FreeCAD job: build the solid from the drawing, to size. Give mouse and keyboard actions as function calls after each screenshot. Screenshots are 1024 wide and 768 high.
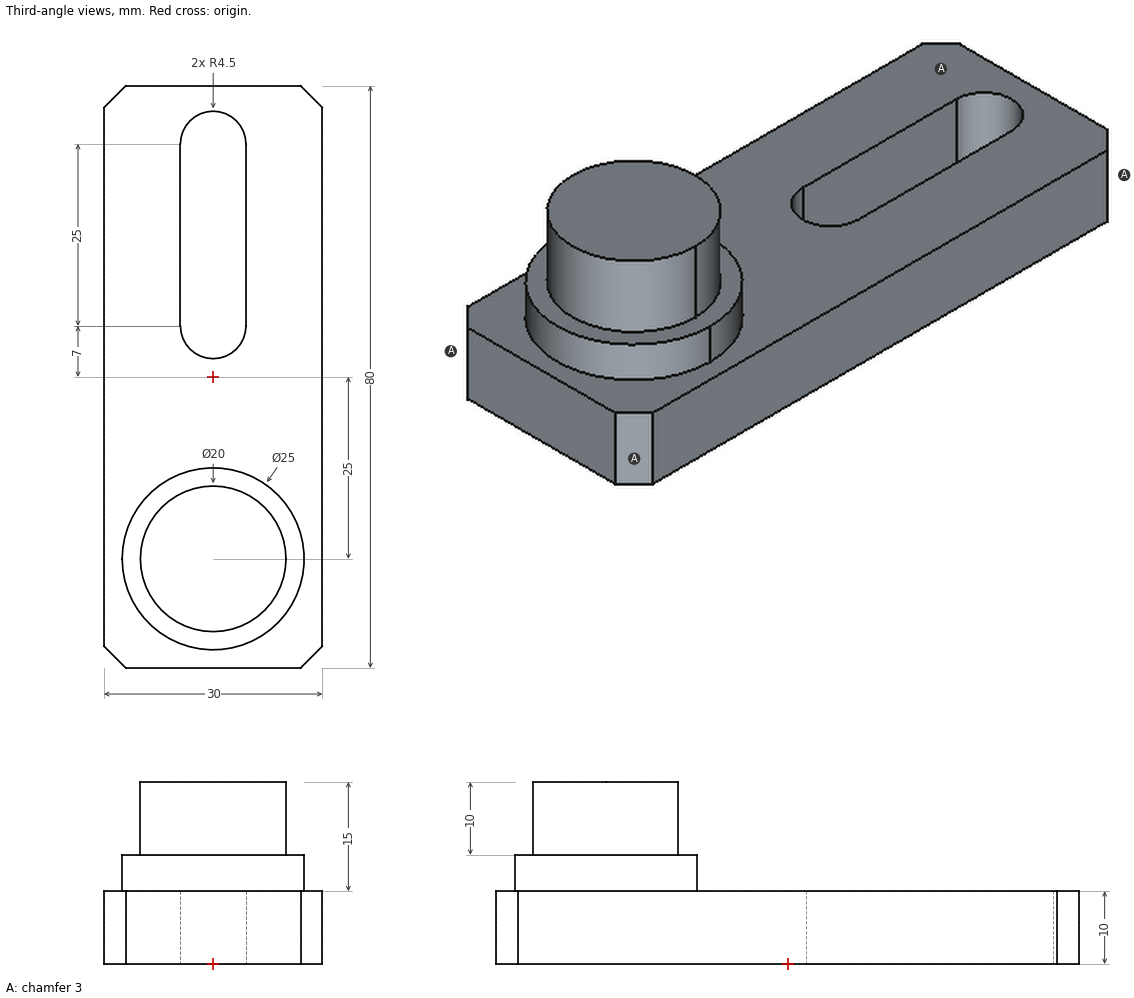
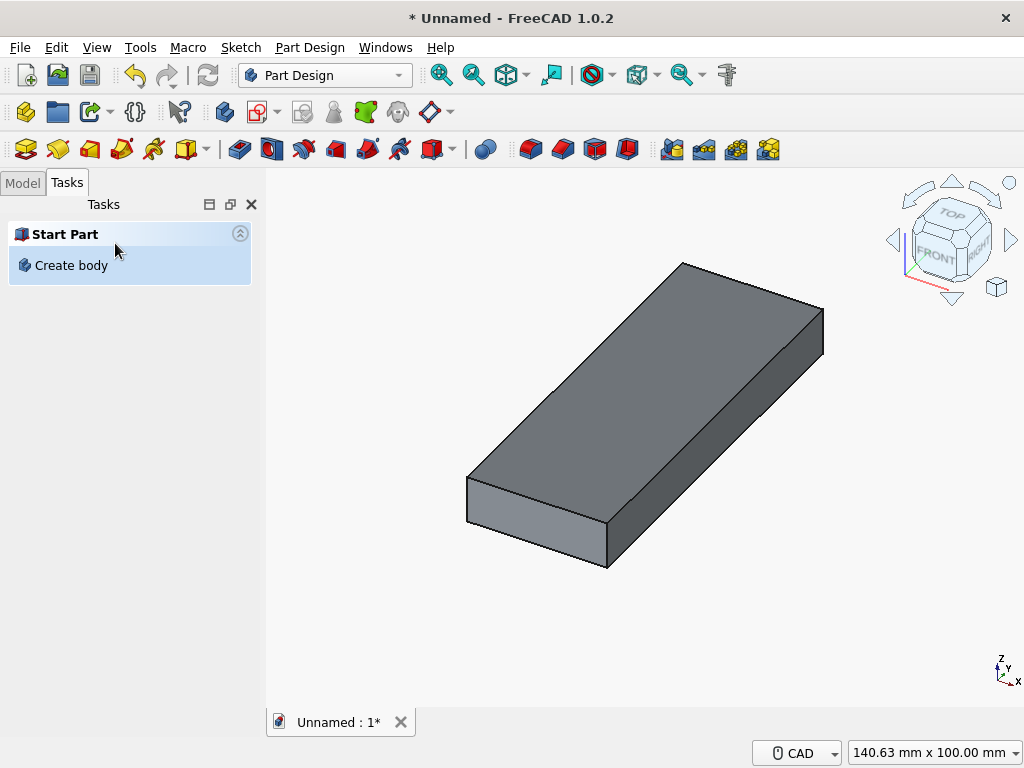
click(707, 331)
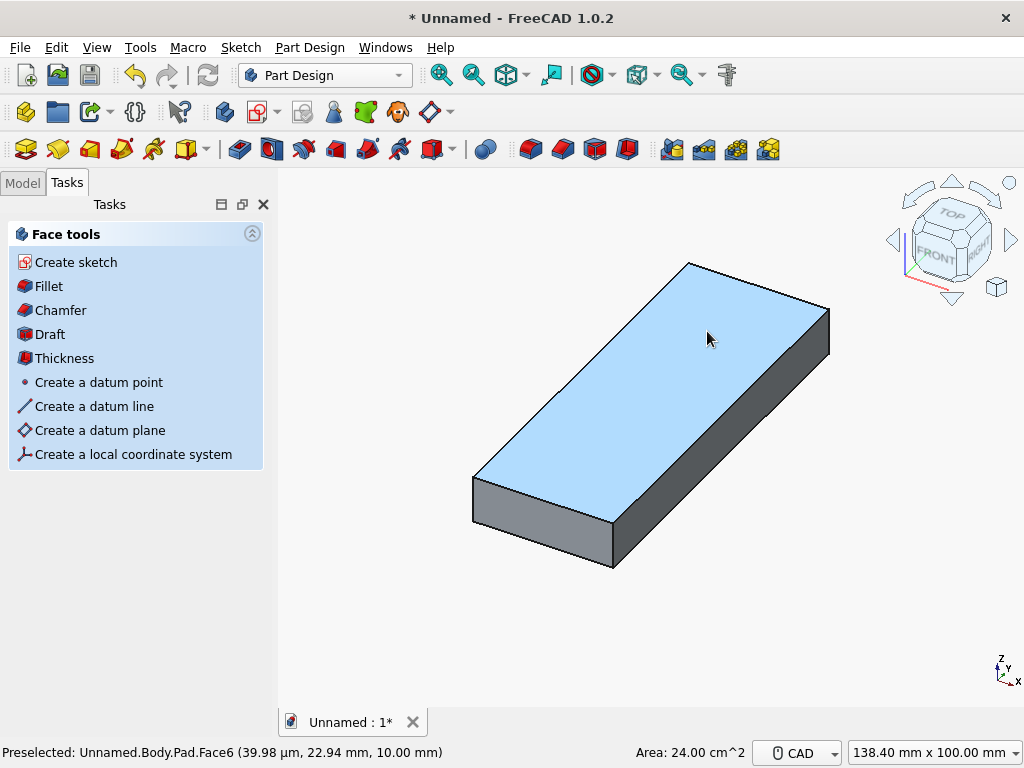
click(258, 112)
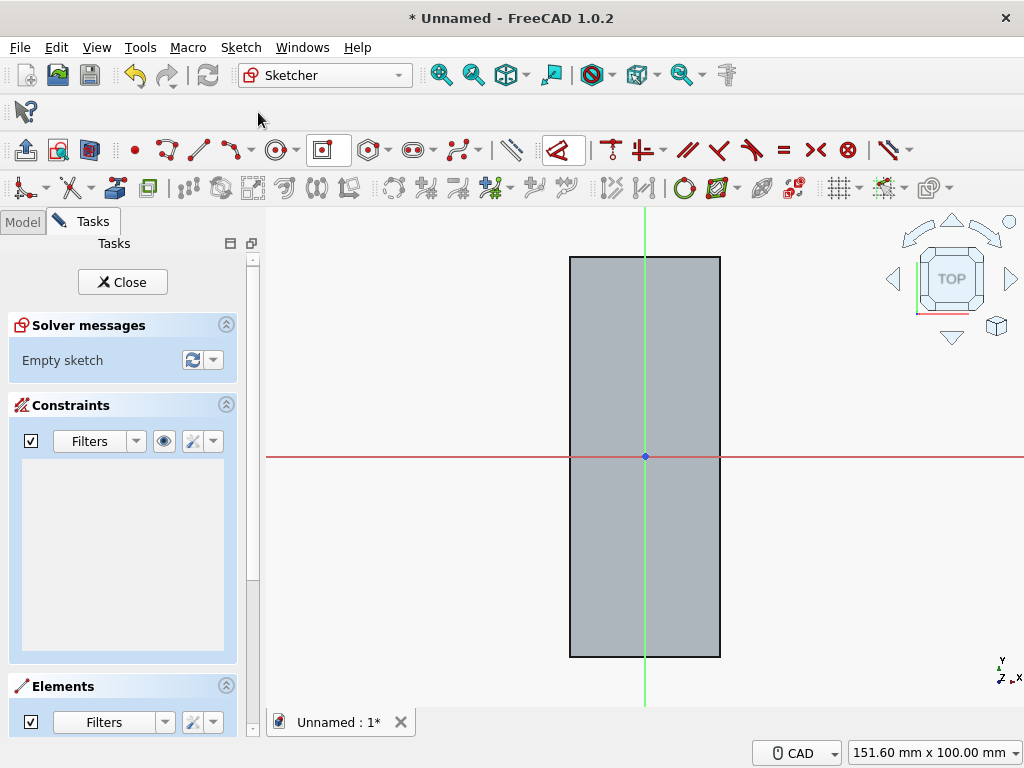
scroll(728, 665, up, 3)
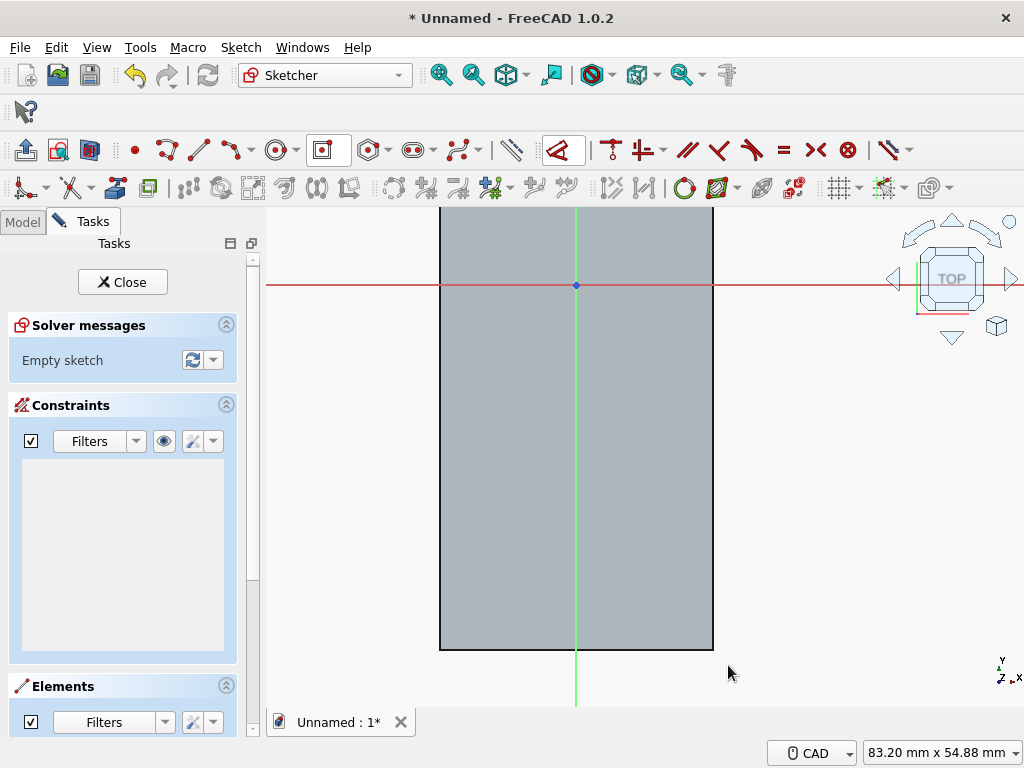
click(276, 150)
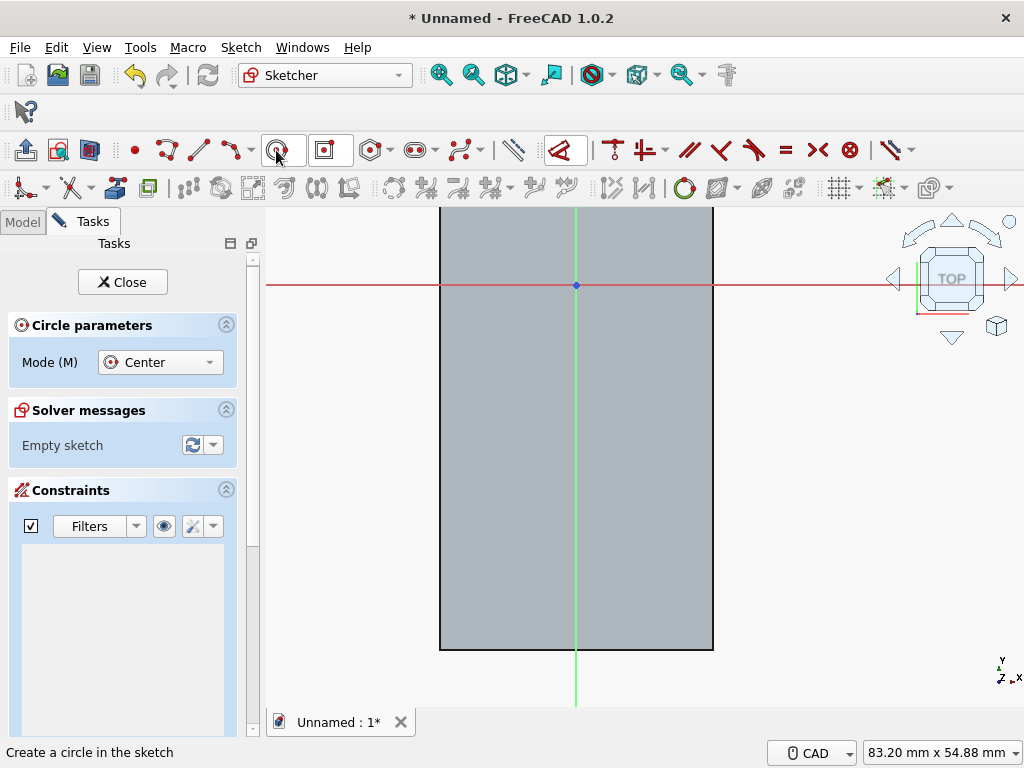
click(576, 513)
move(657, 432)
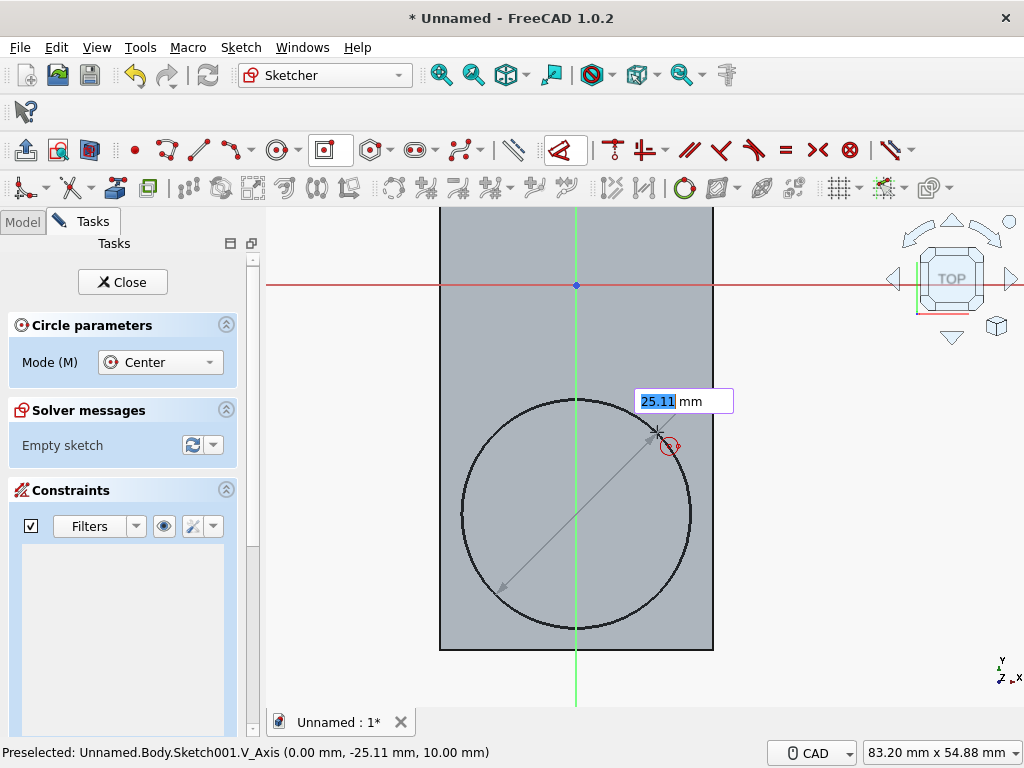
text(25)
key(Return)
key(Escape)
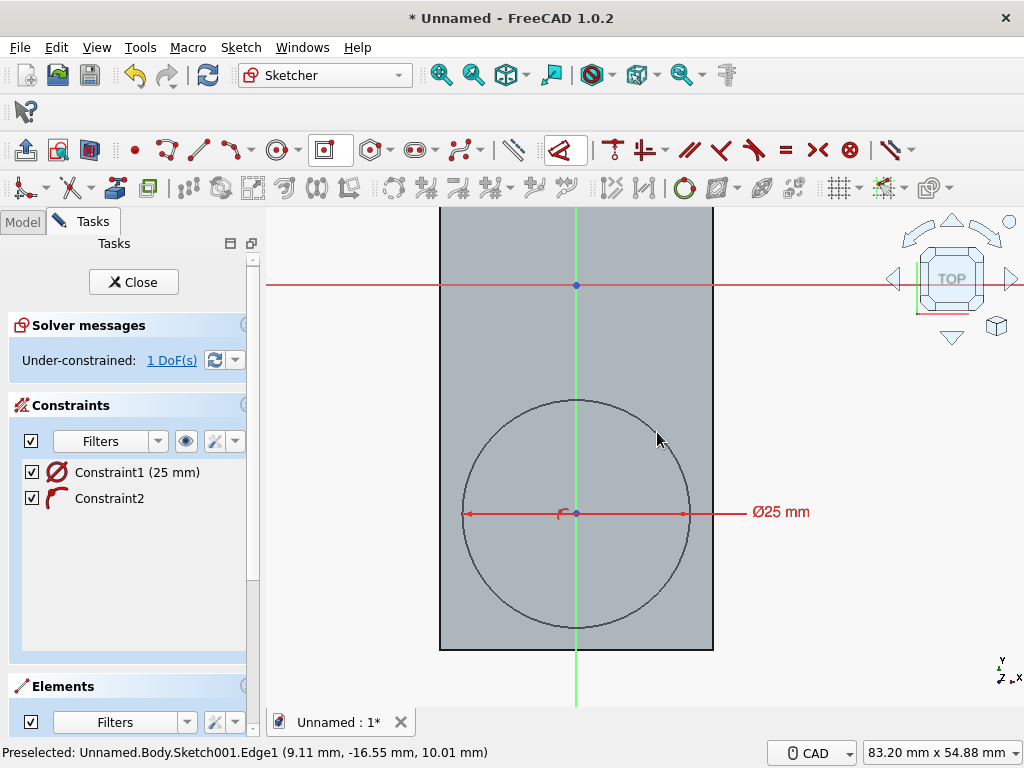
click(560, 150)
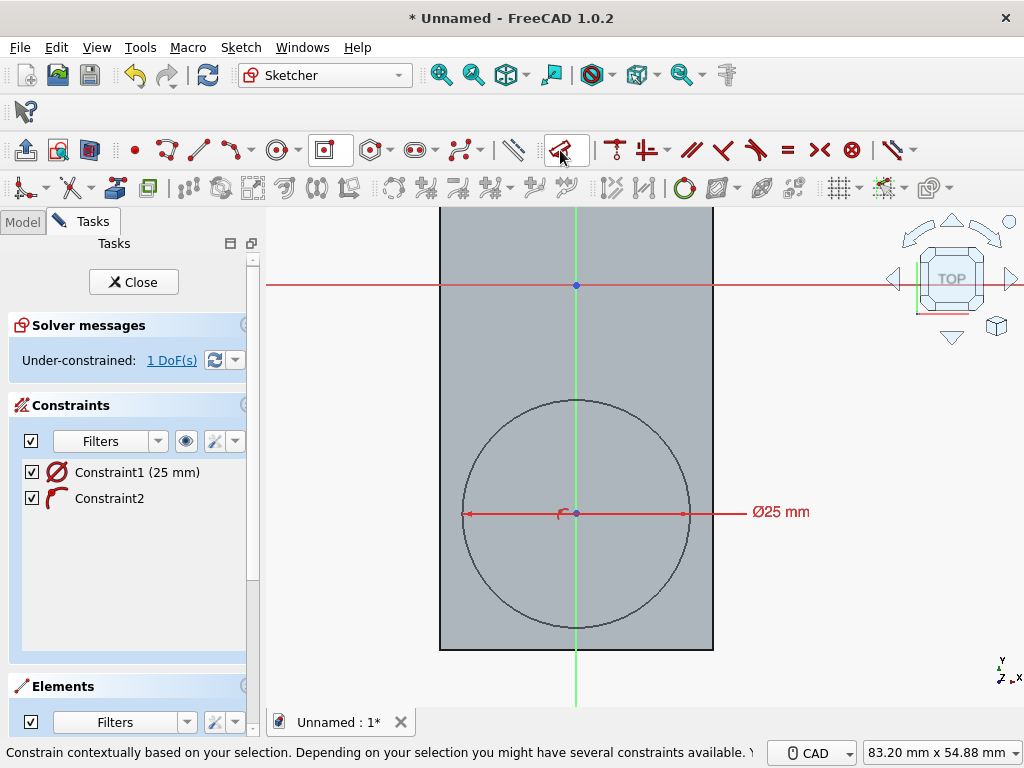
click(576, 514)
click(610, 347)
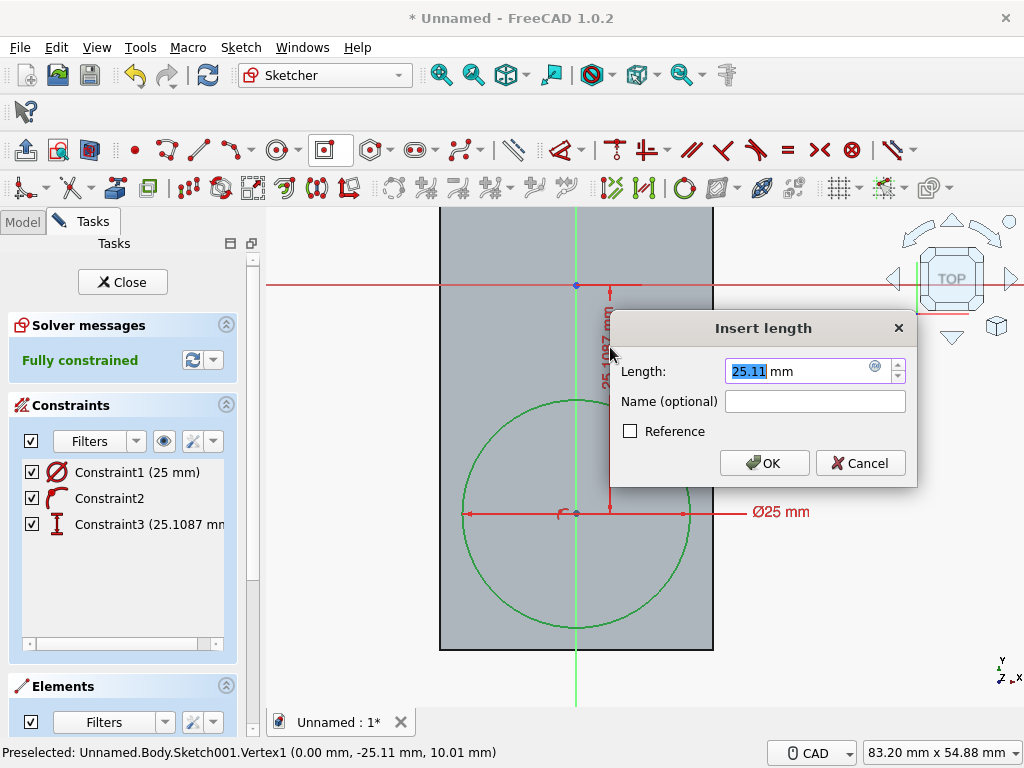
text(25)
key(Return)
key(Escape)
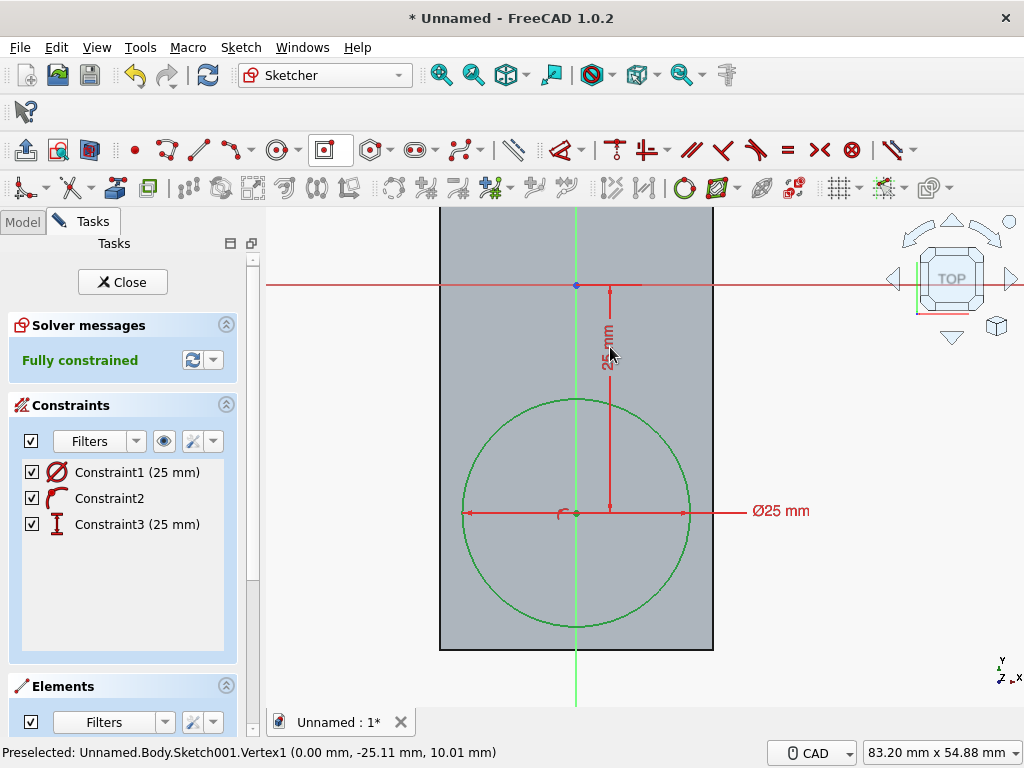
click(123, 282)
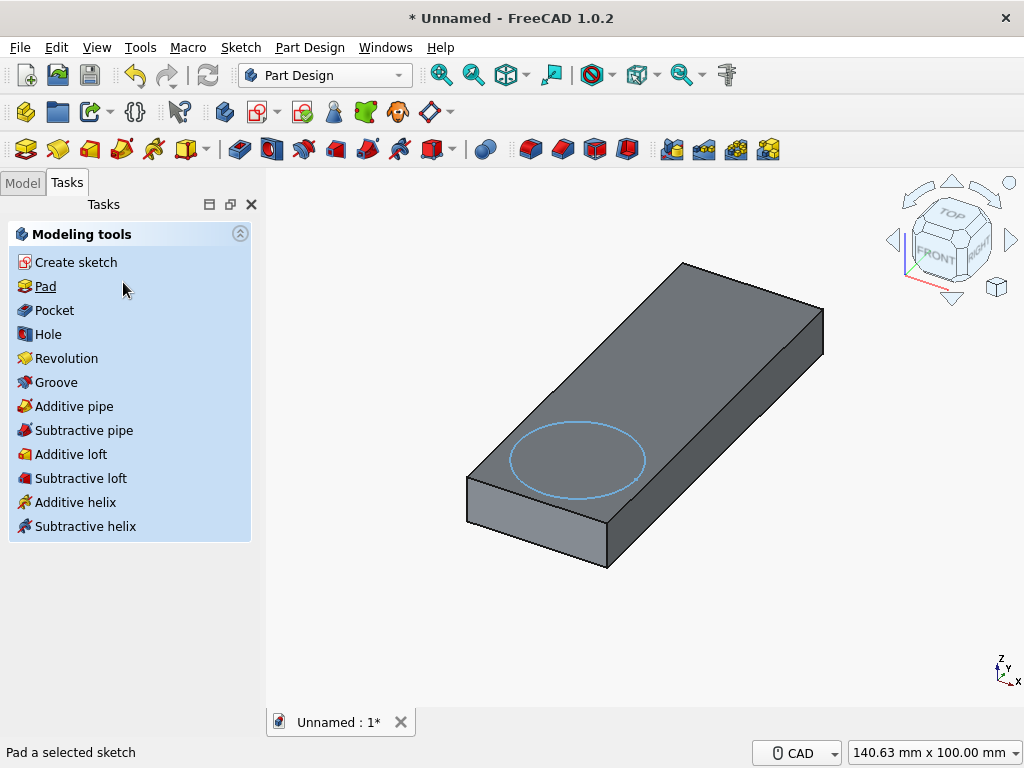
click(26, 150)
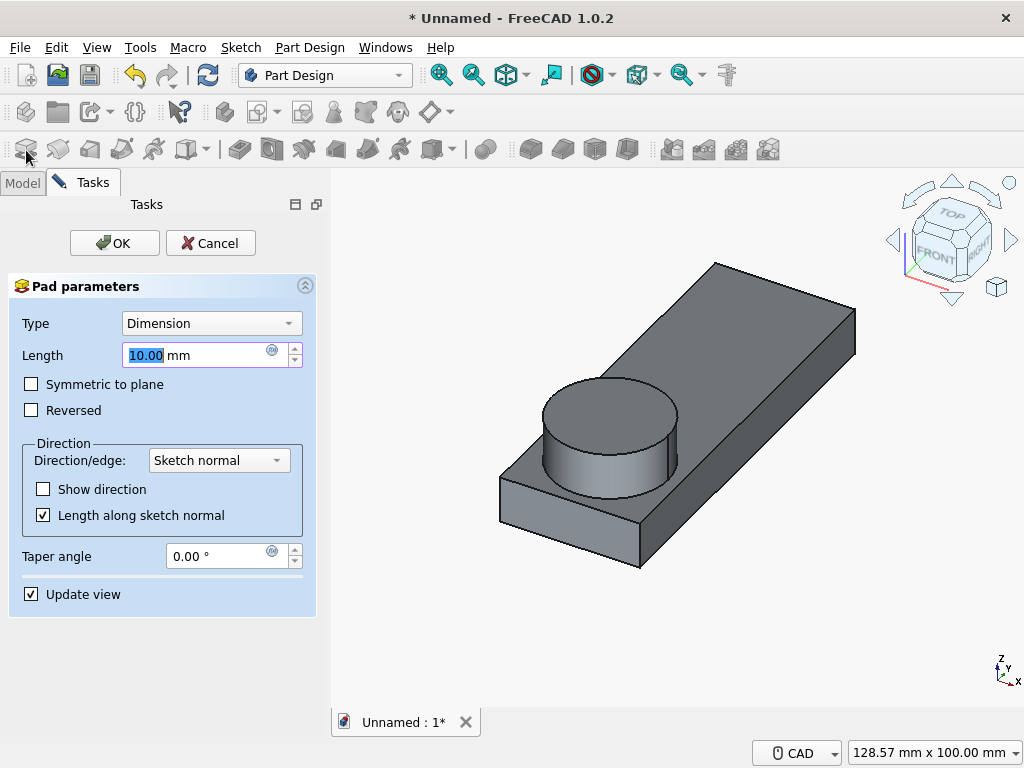
text(15)
key(Tab)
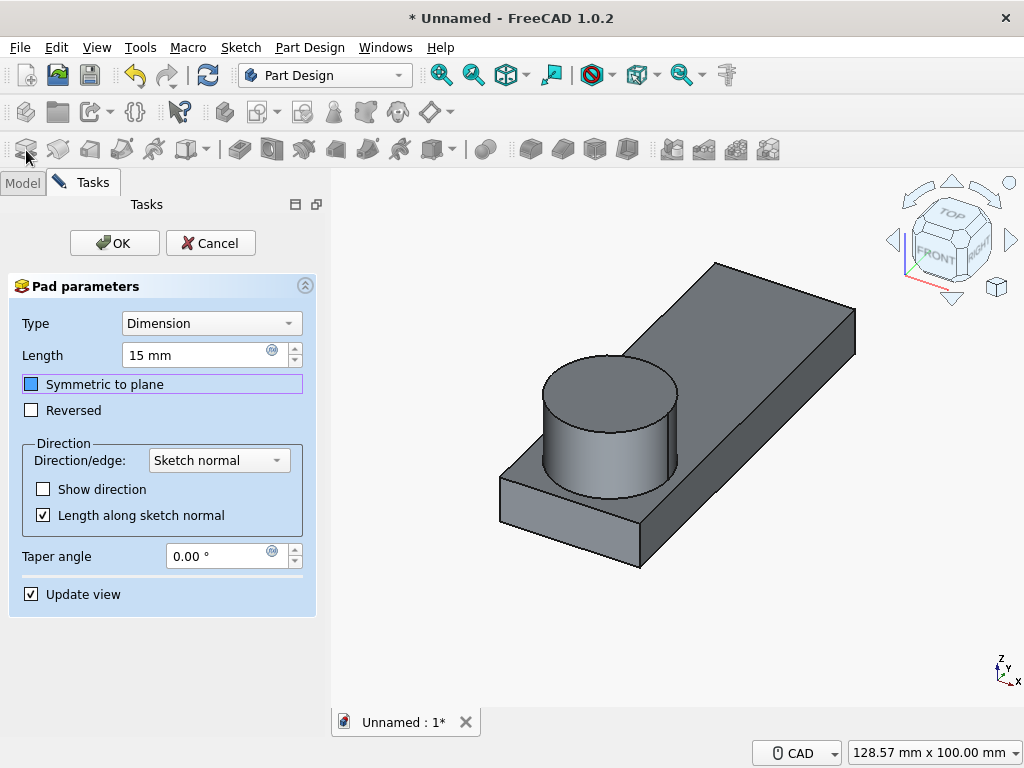
click(115, 243)